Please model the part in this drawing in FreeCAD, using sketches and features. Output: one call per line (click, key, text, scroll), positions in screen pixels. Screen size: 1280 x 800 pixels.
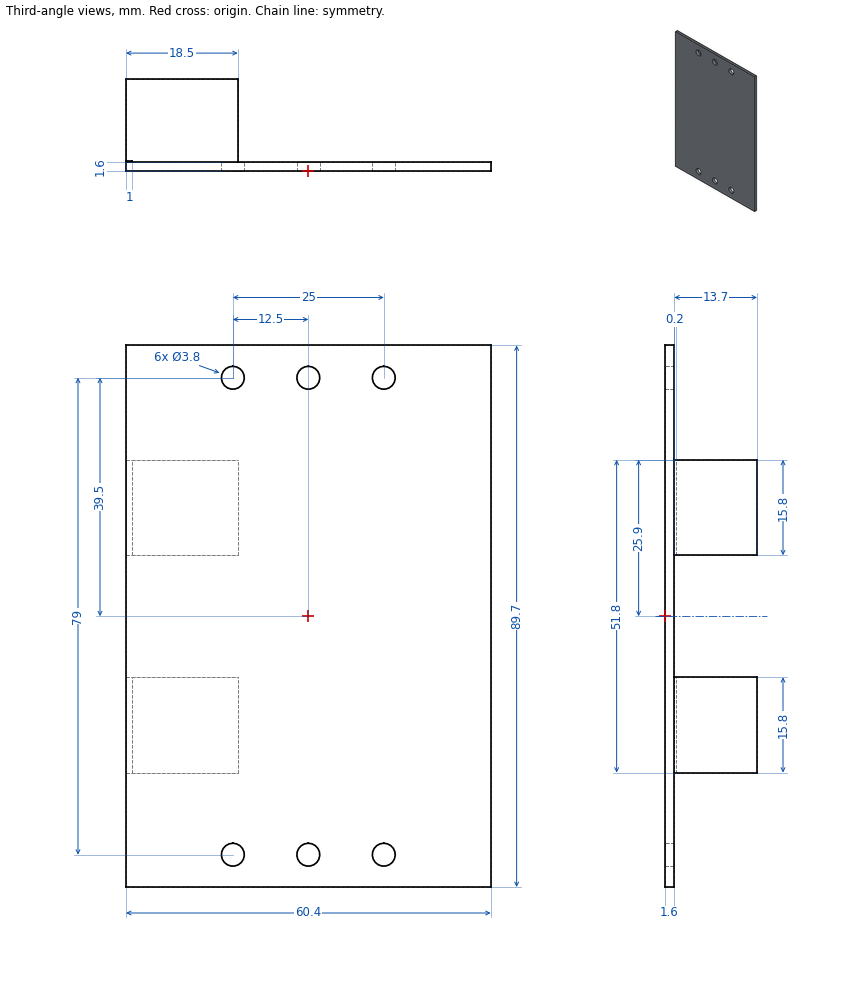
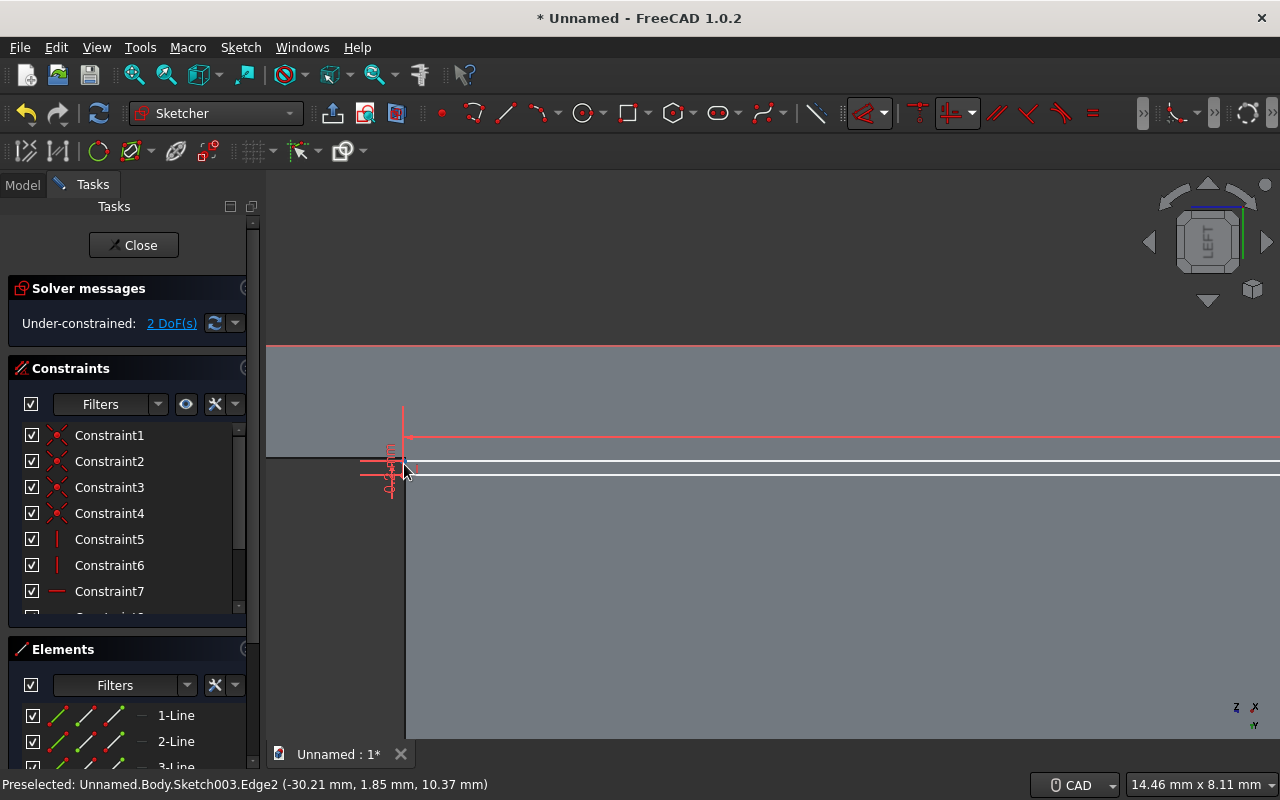
click(403, 461)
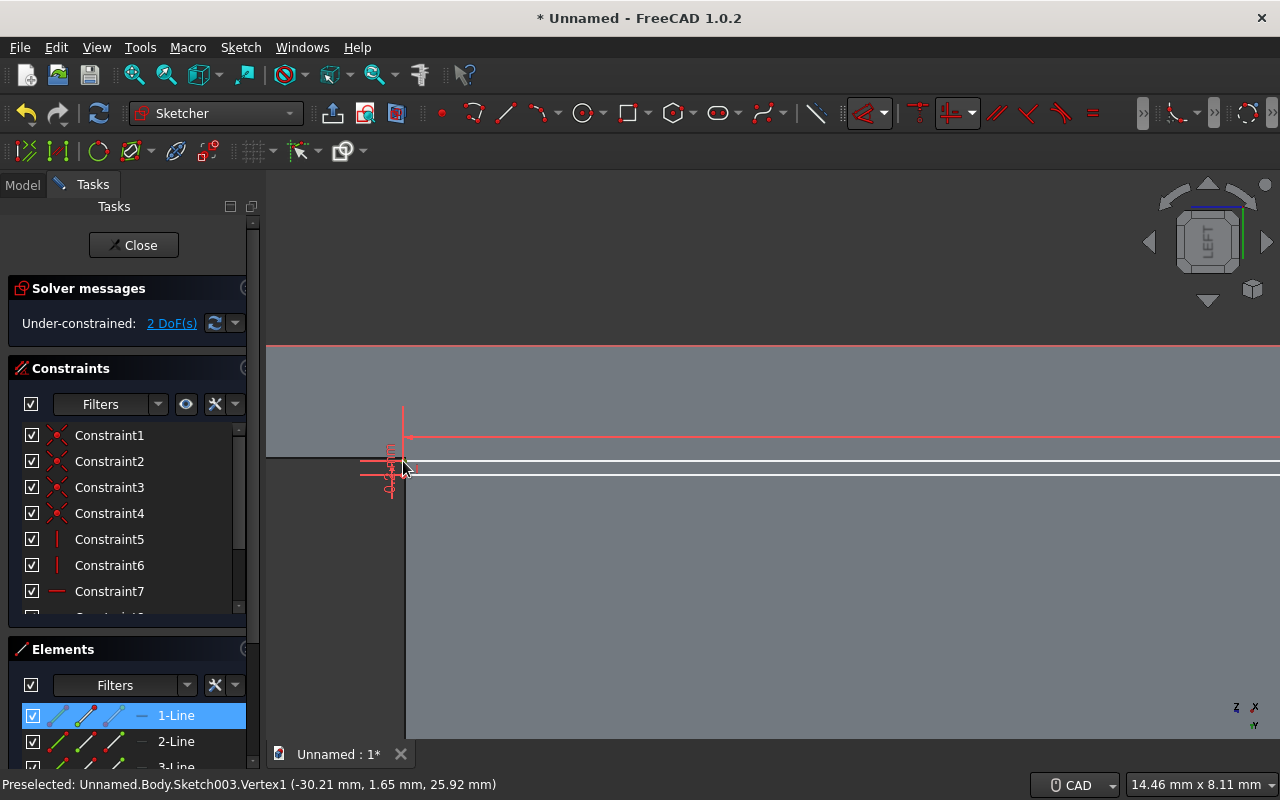
key(i)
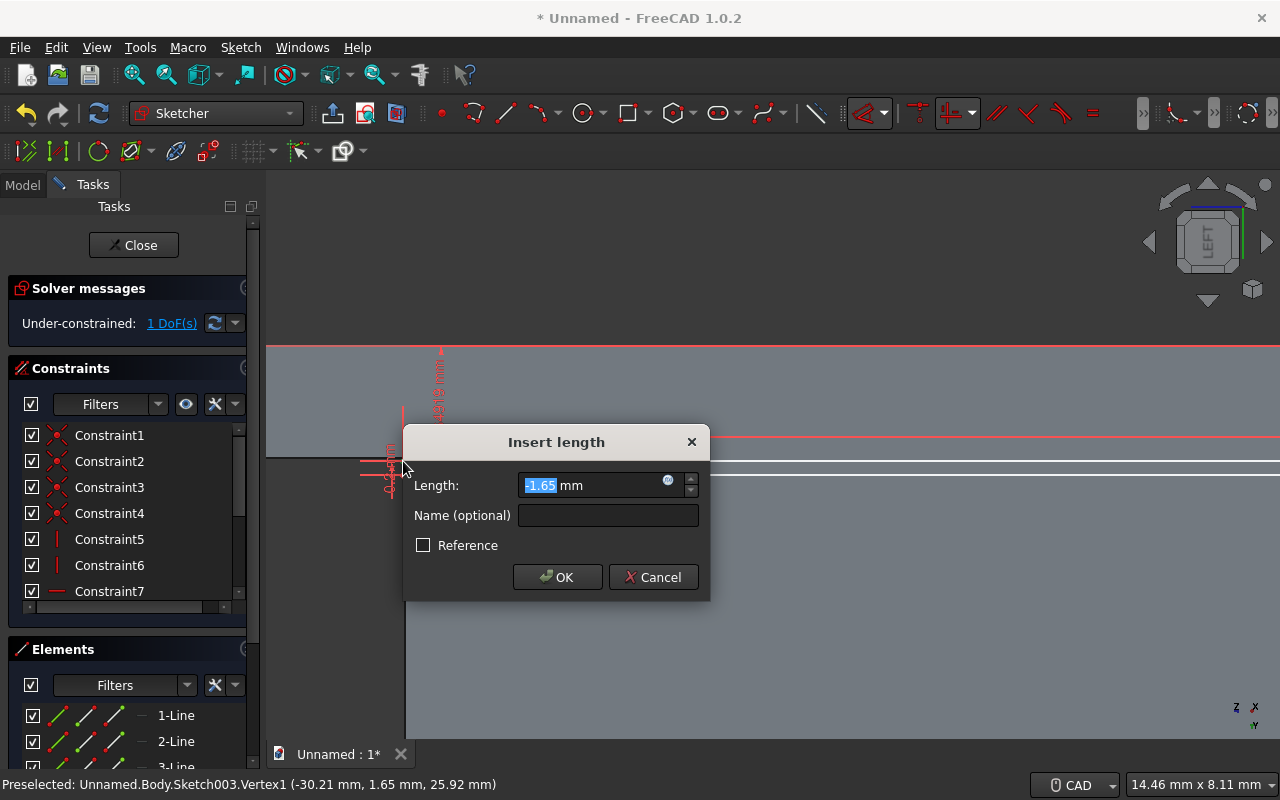
text(-1.6)
key(Return)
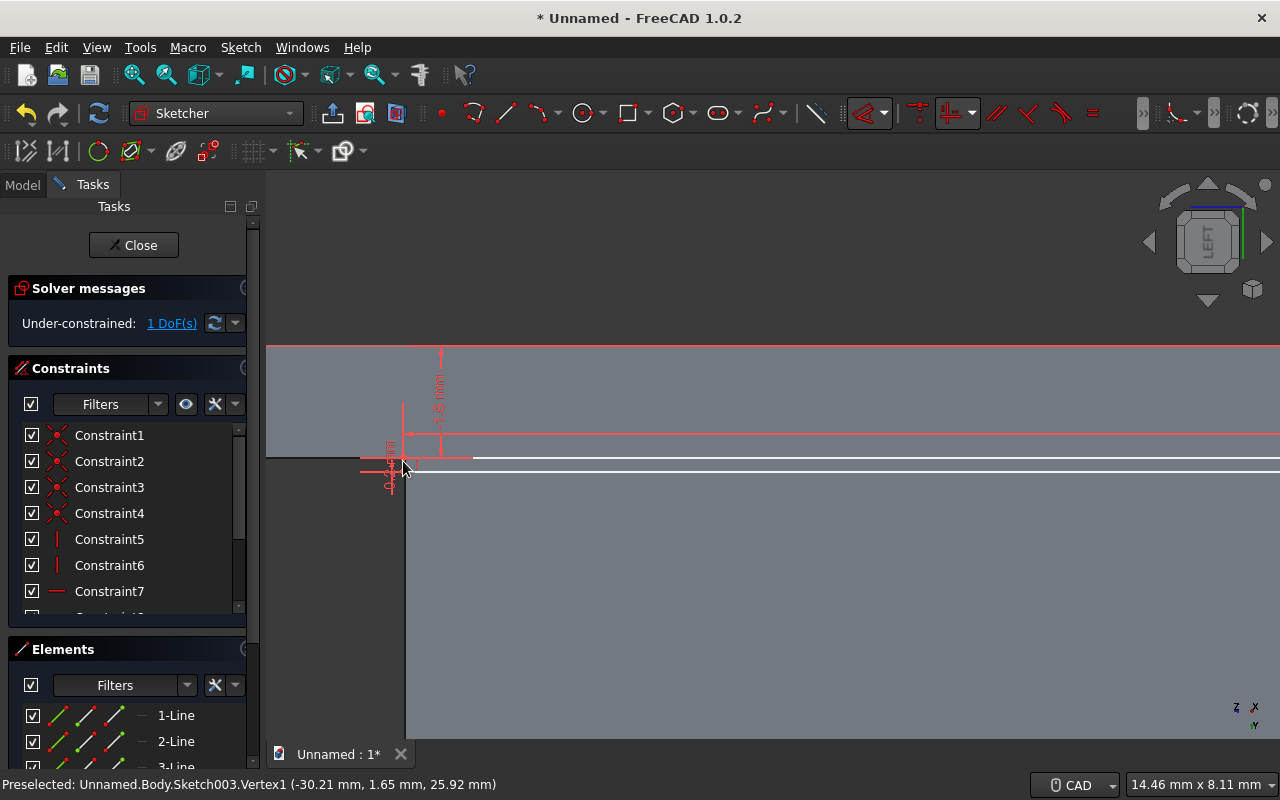
click(403, 458)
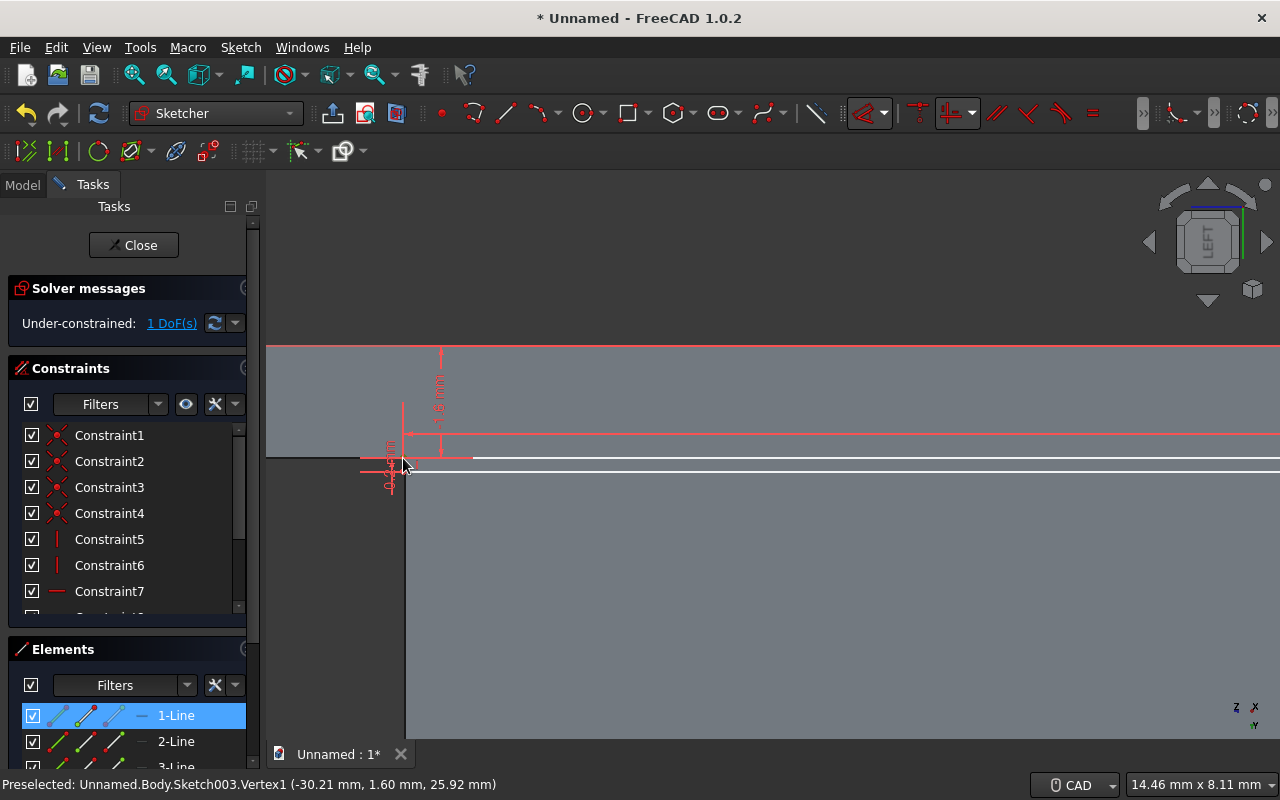
key(l)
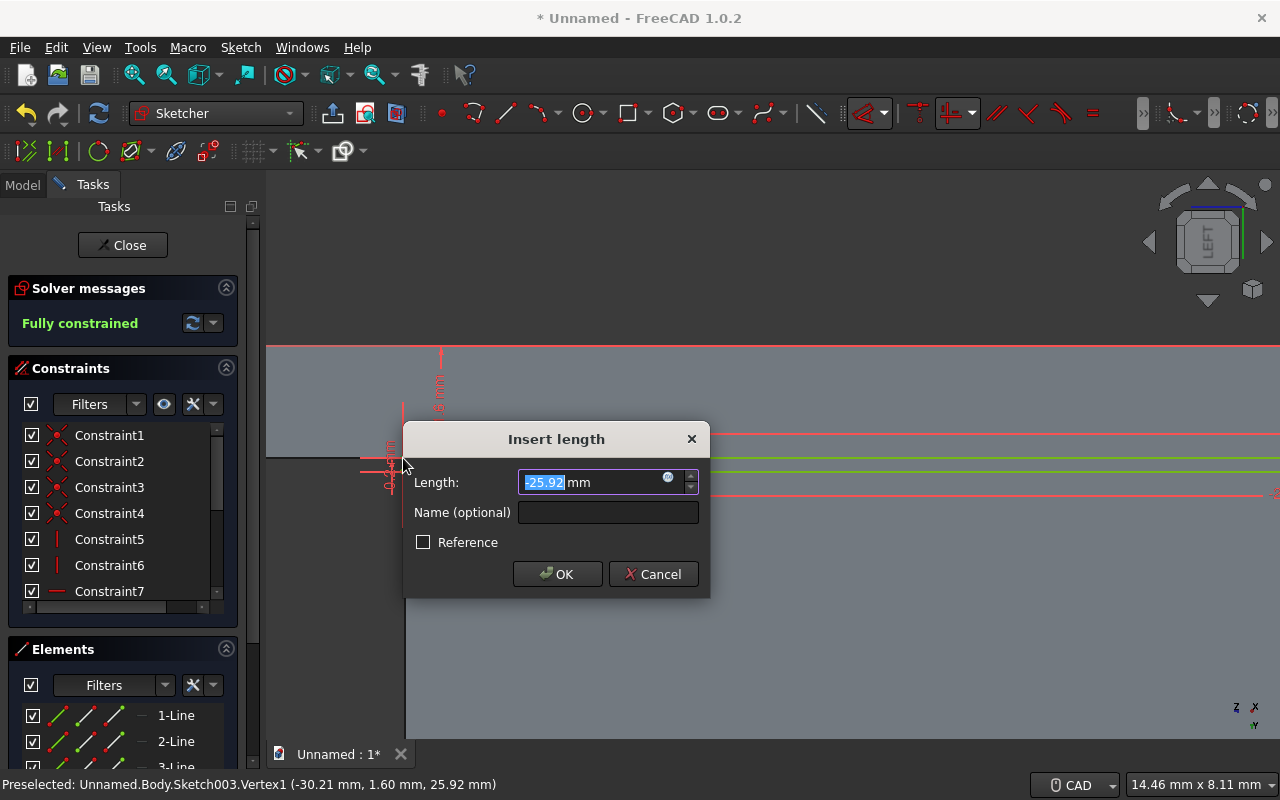
text(-25.9)
key(Return)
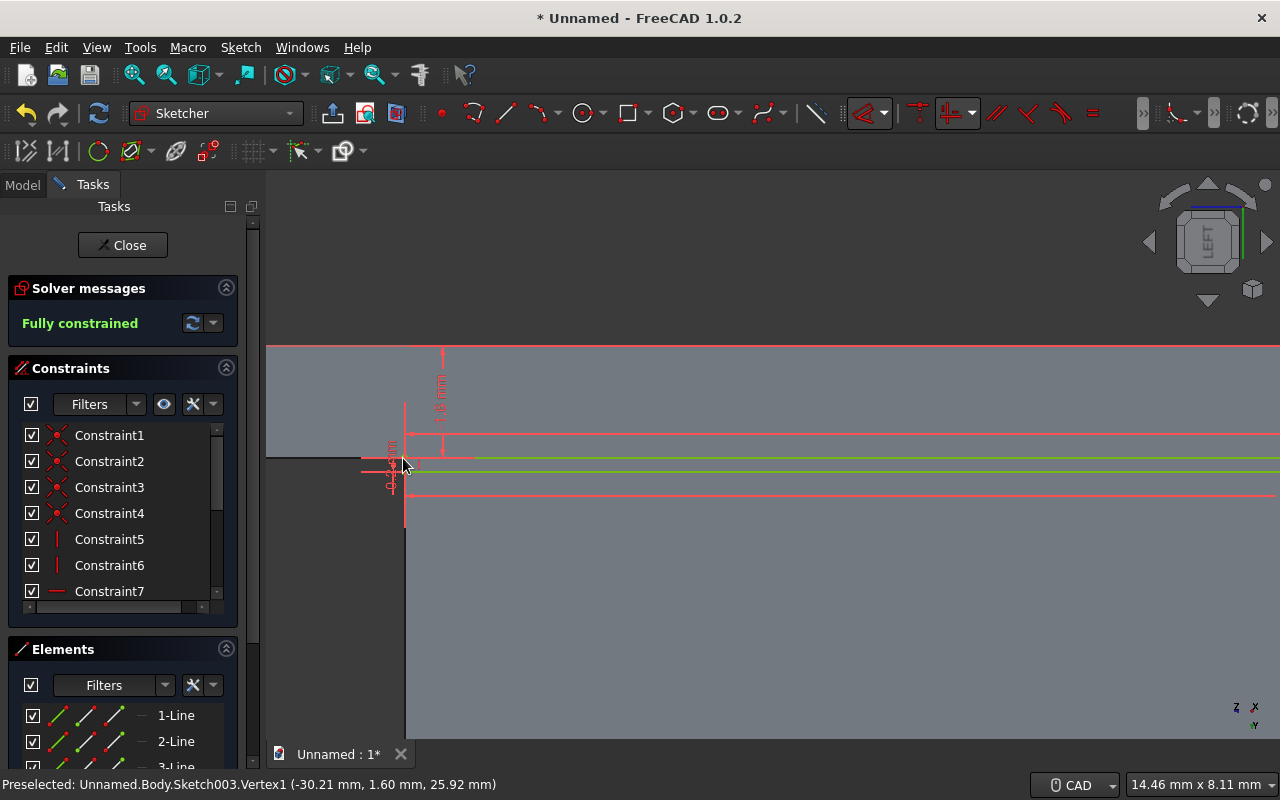
click(123, 245)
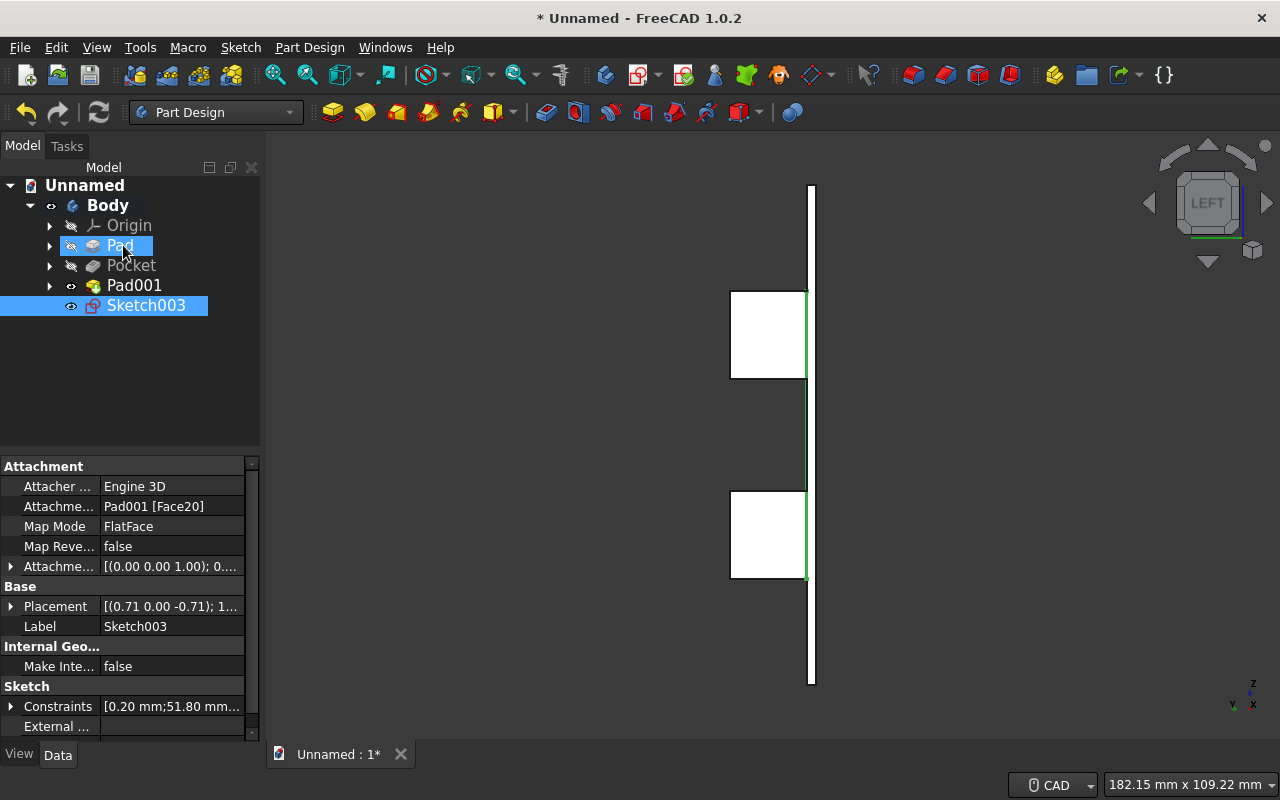
click(548, 112)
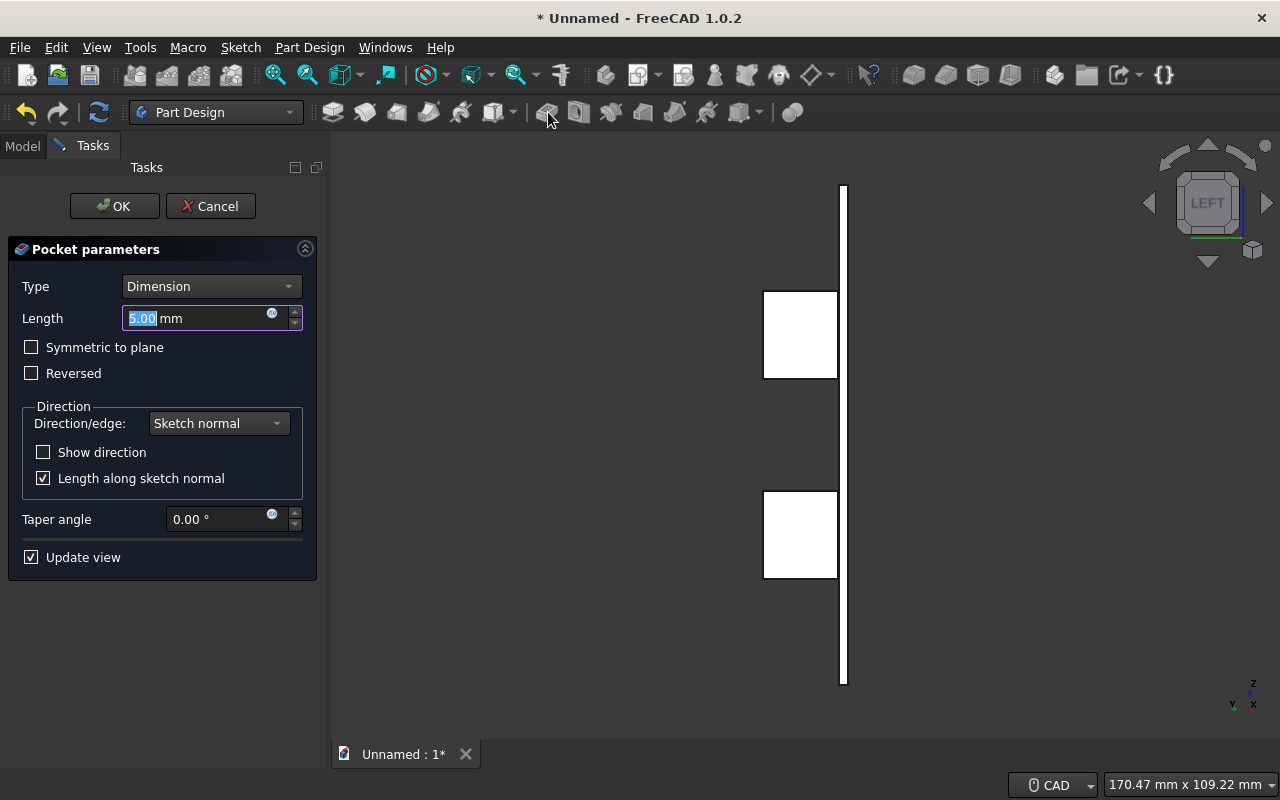
text(1)
key(Tab)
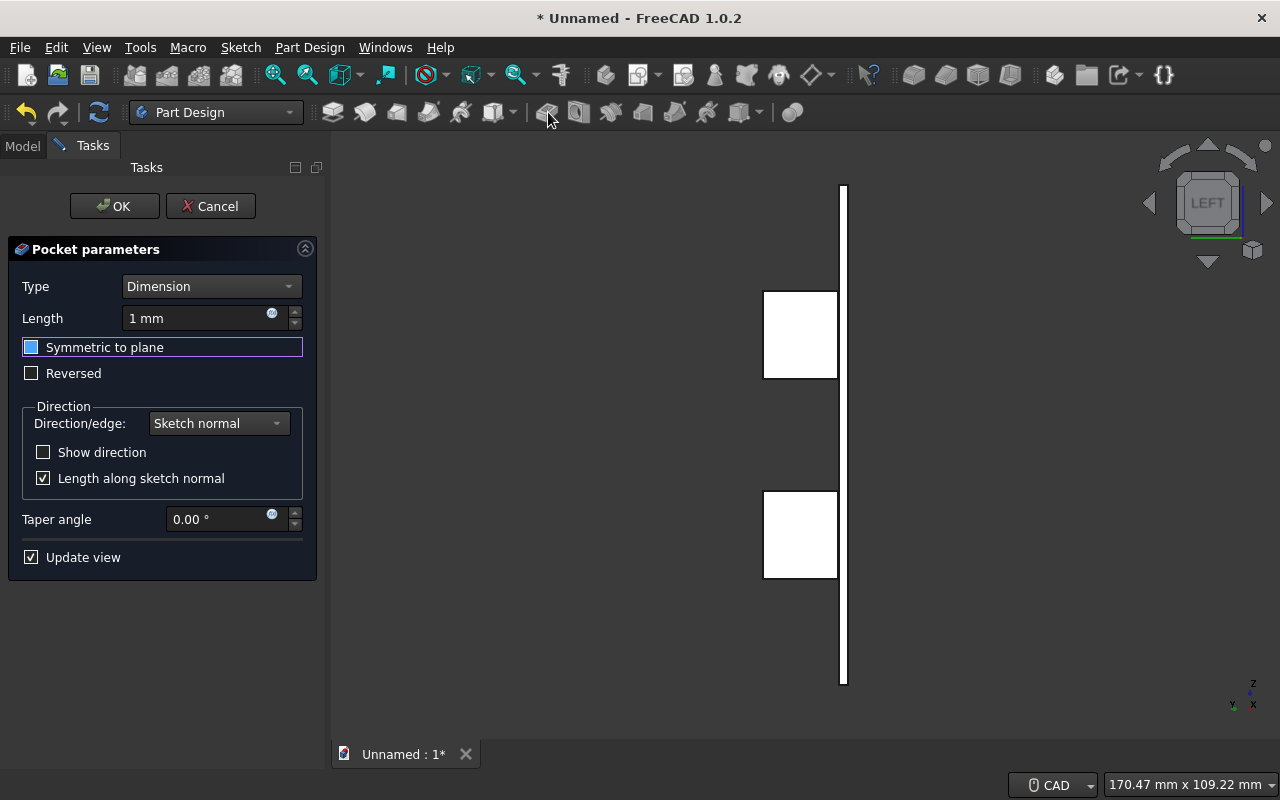
click(115, 206)